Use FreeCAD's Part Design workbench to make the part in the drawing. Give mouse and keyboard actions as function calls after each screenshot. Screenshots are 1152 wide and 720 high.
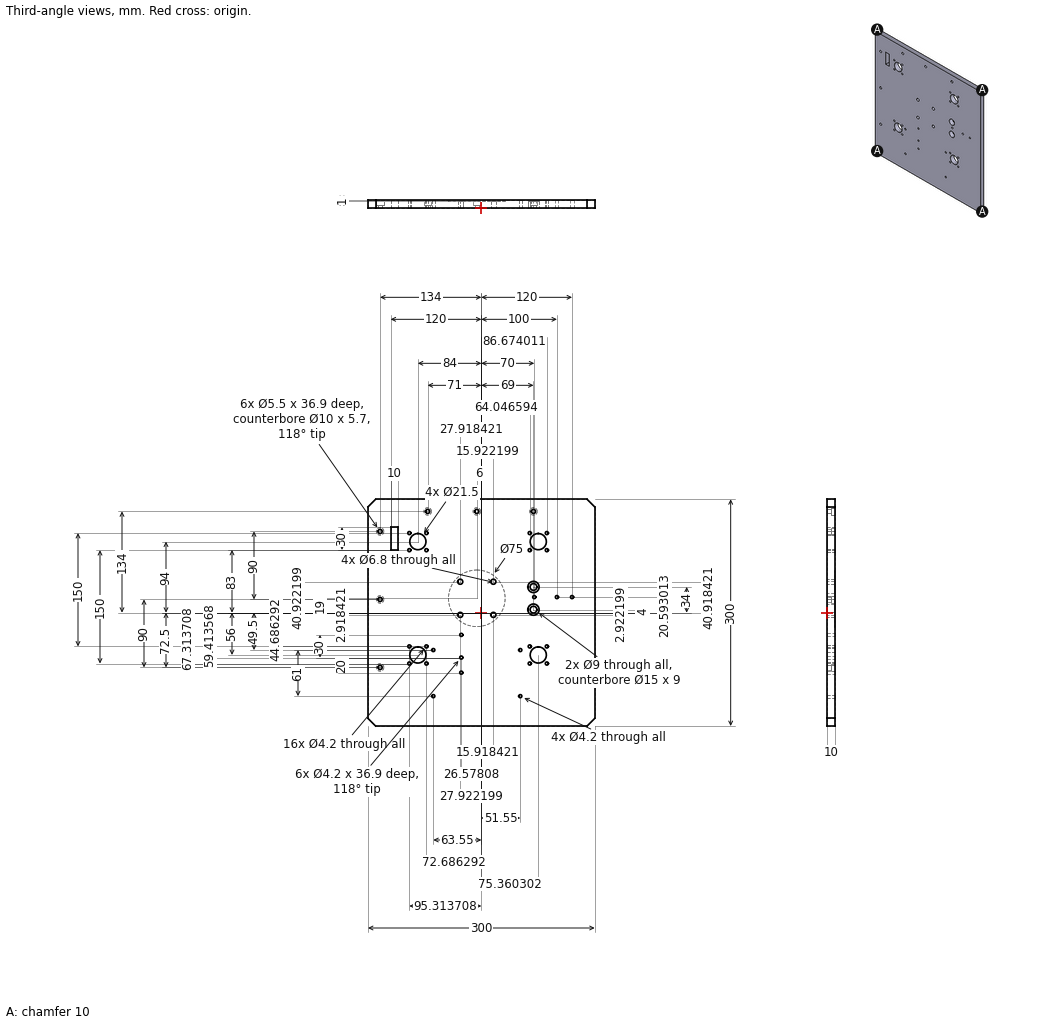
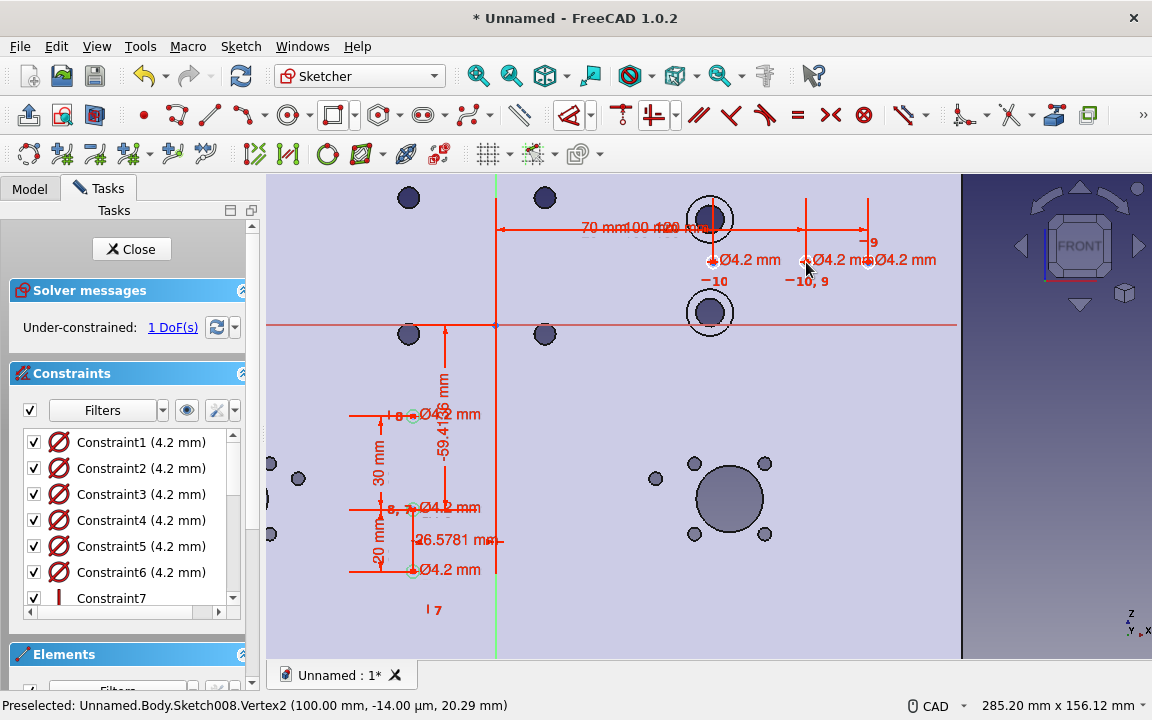
click(590, 116)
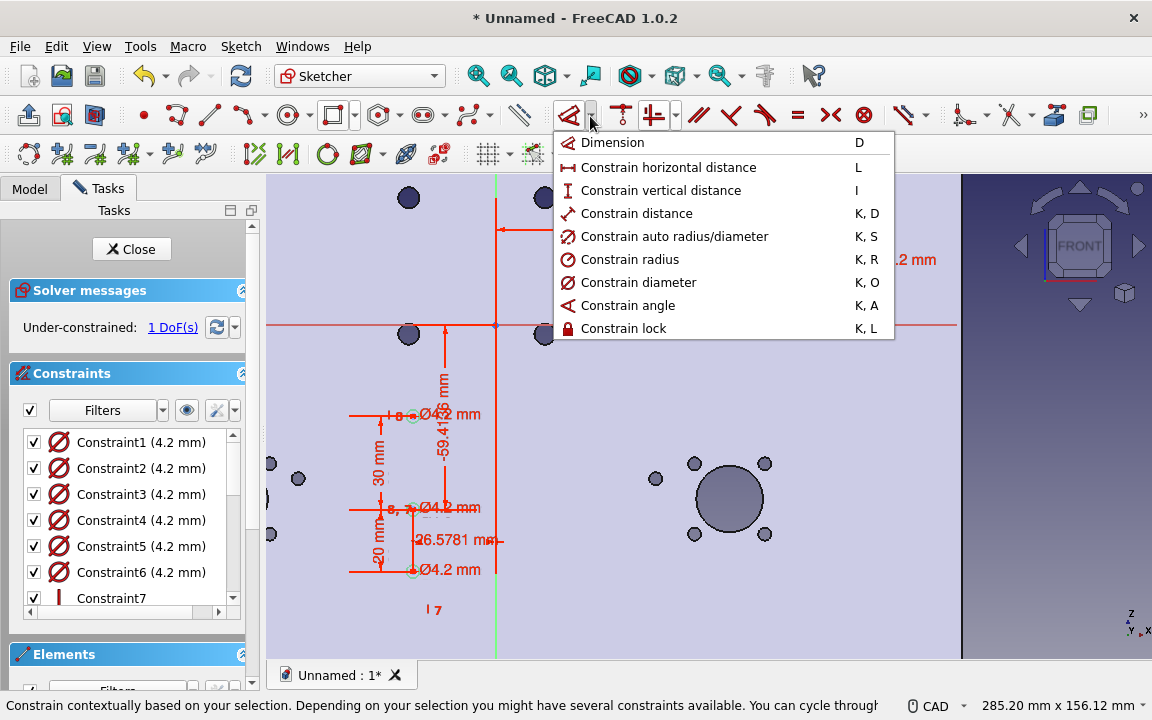
click(724, 190)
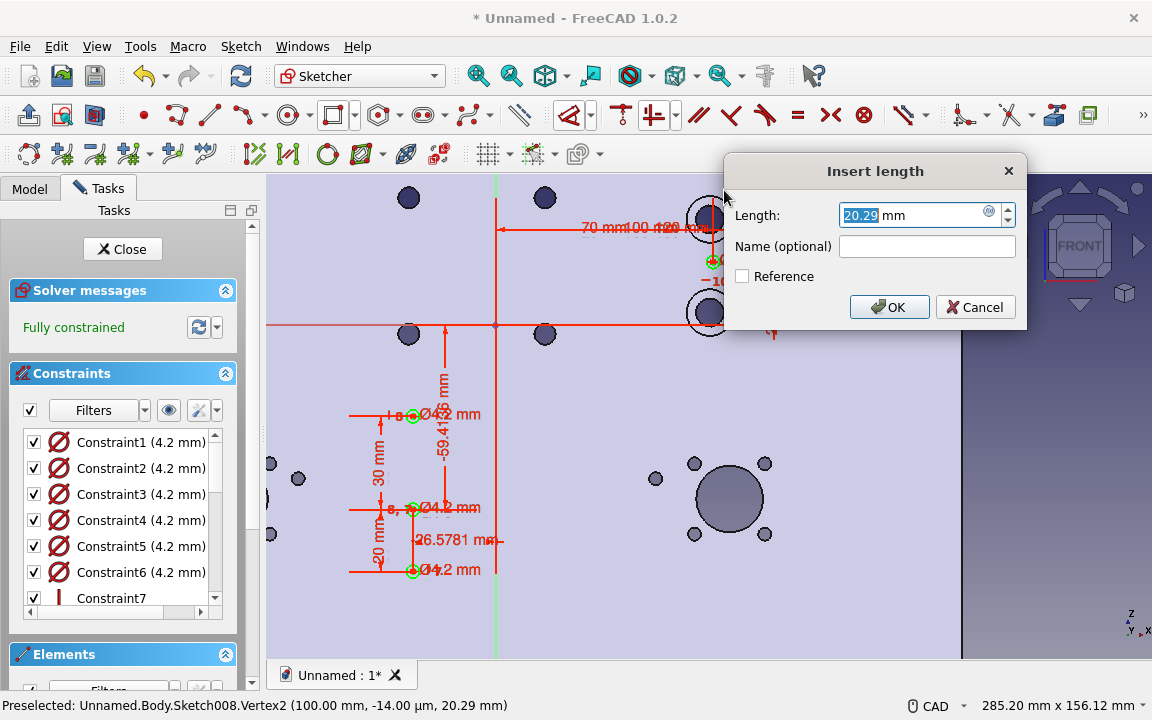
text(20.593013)
key(Return)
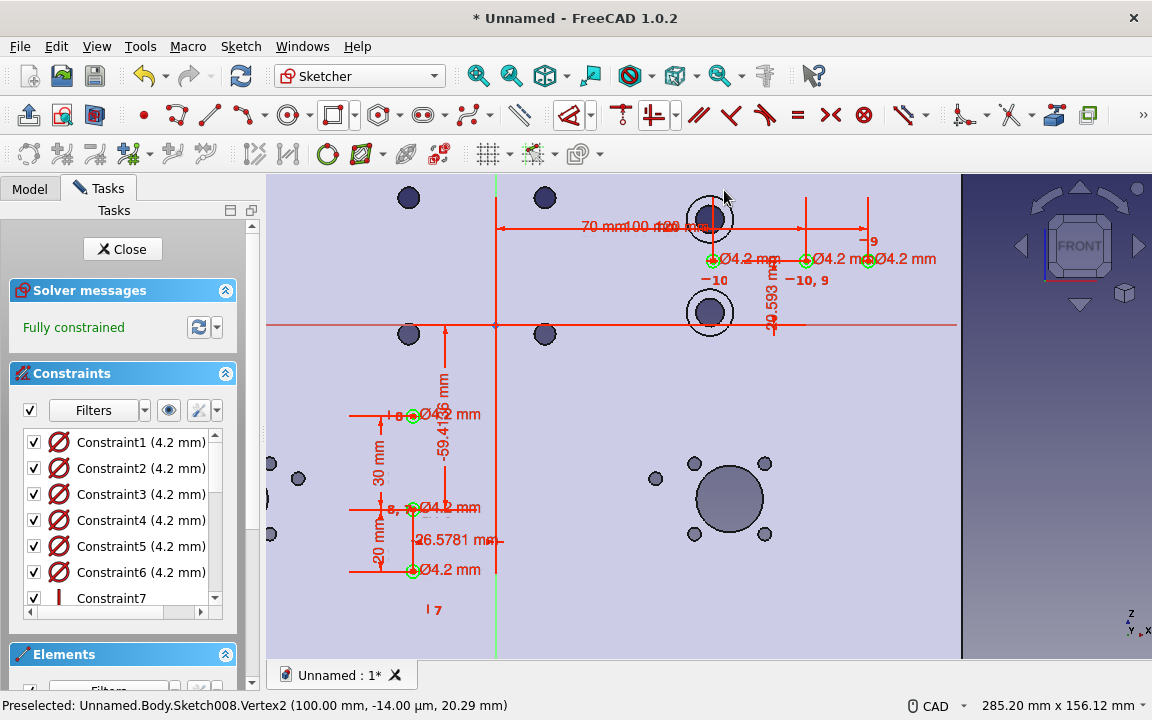
click(123, 249)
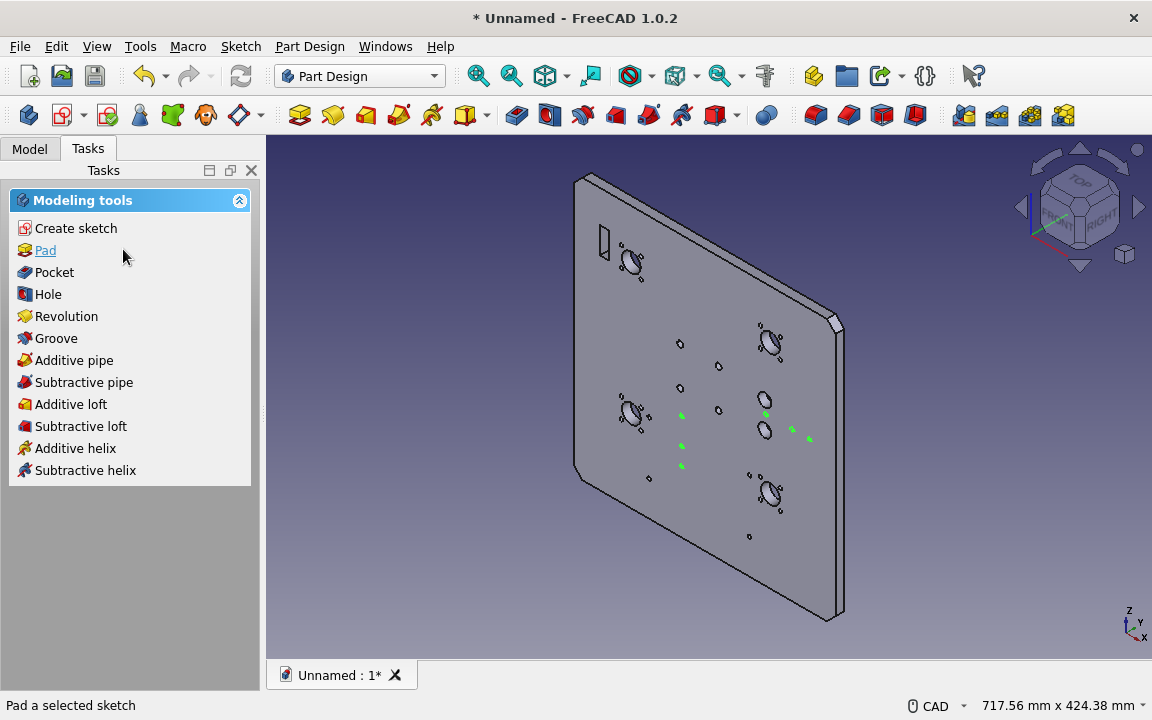
click(550, 116)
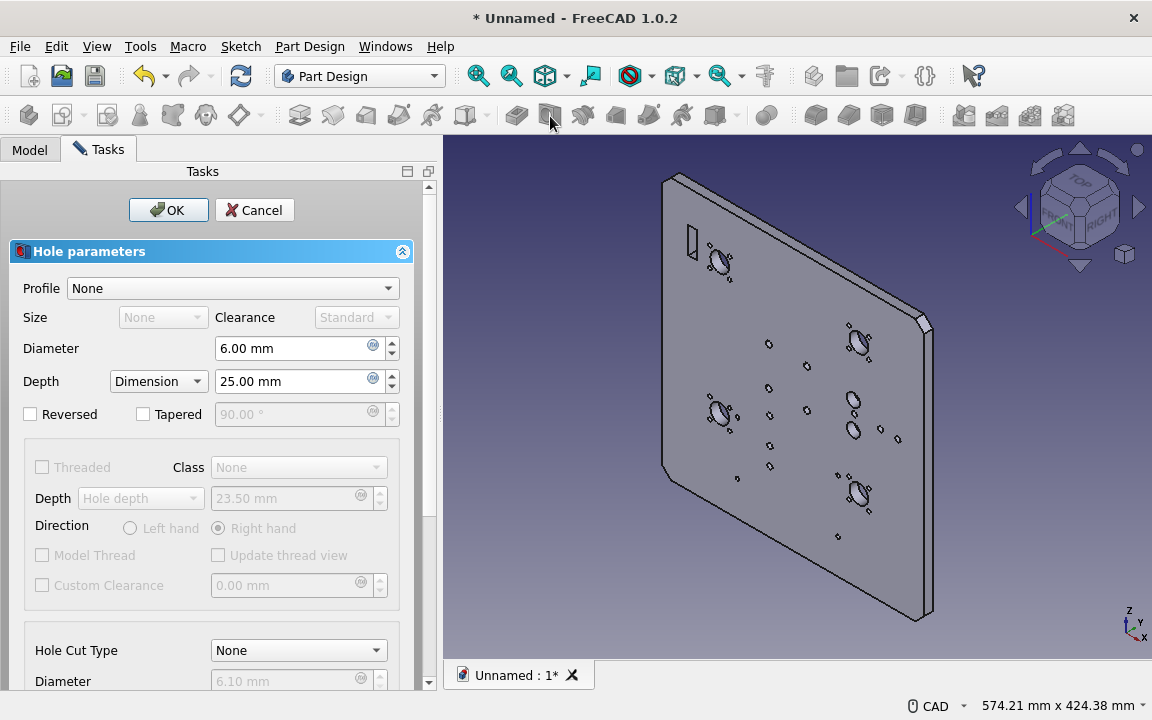
triple_click(300, 348)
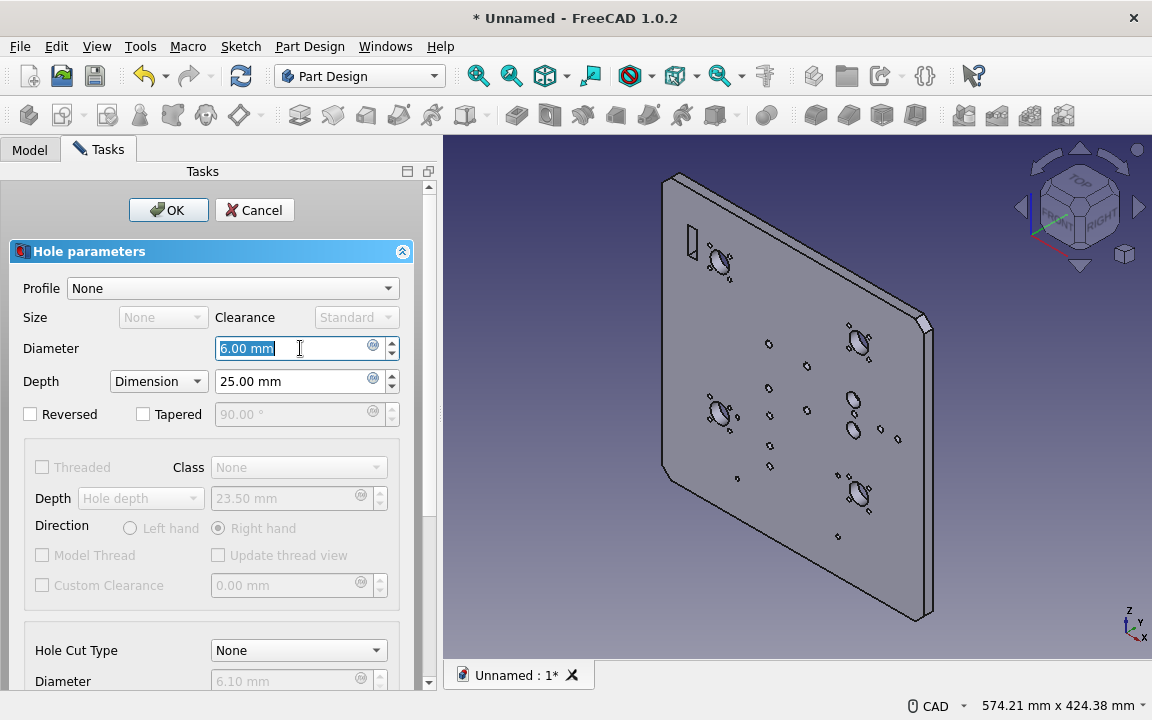
text(4.2)
key(Tab)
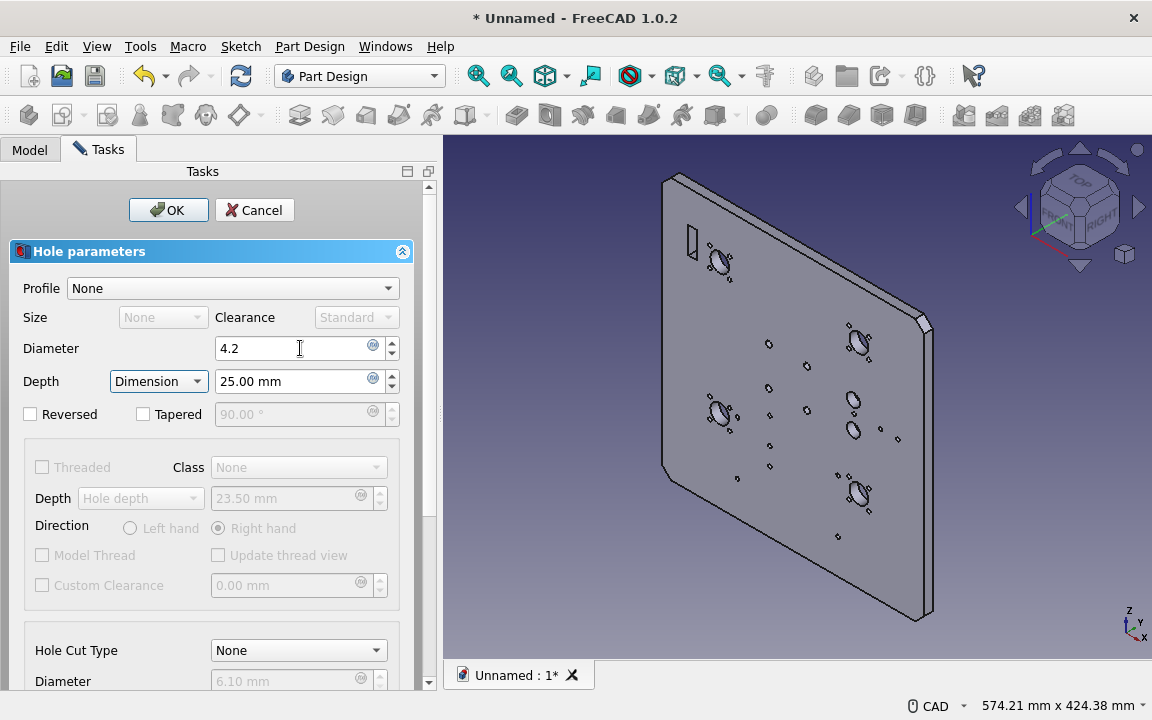
triple_click(300, 382)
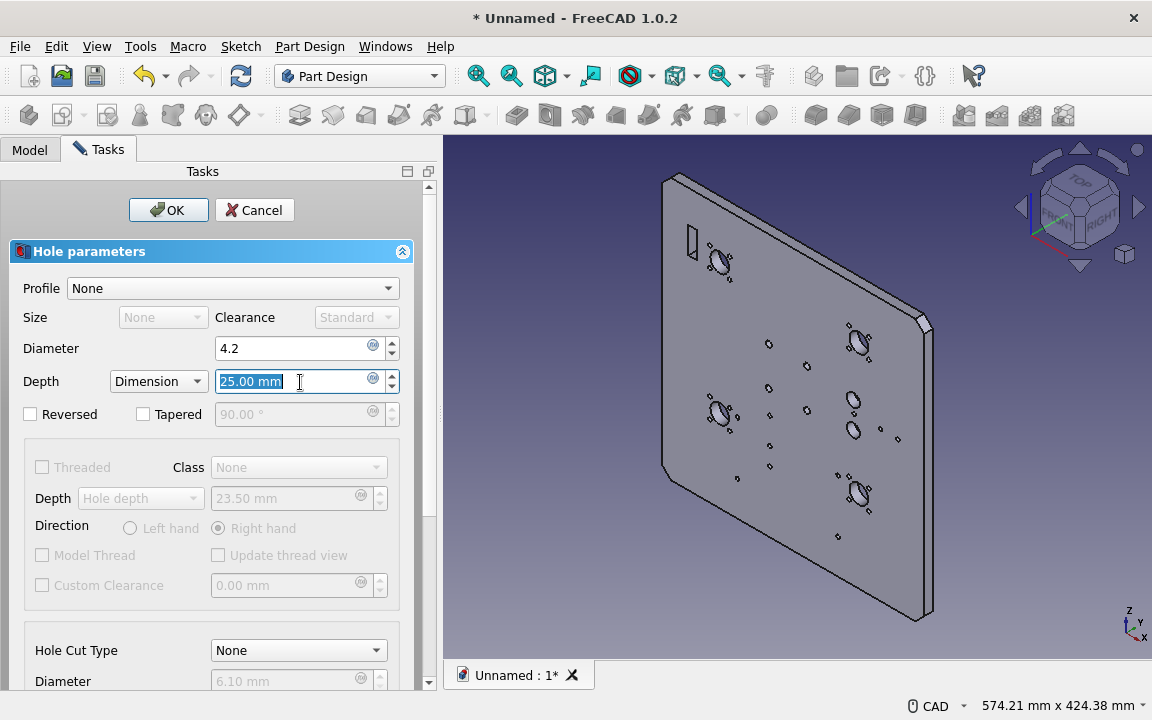
text(36.9)
key(Tab)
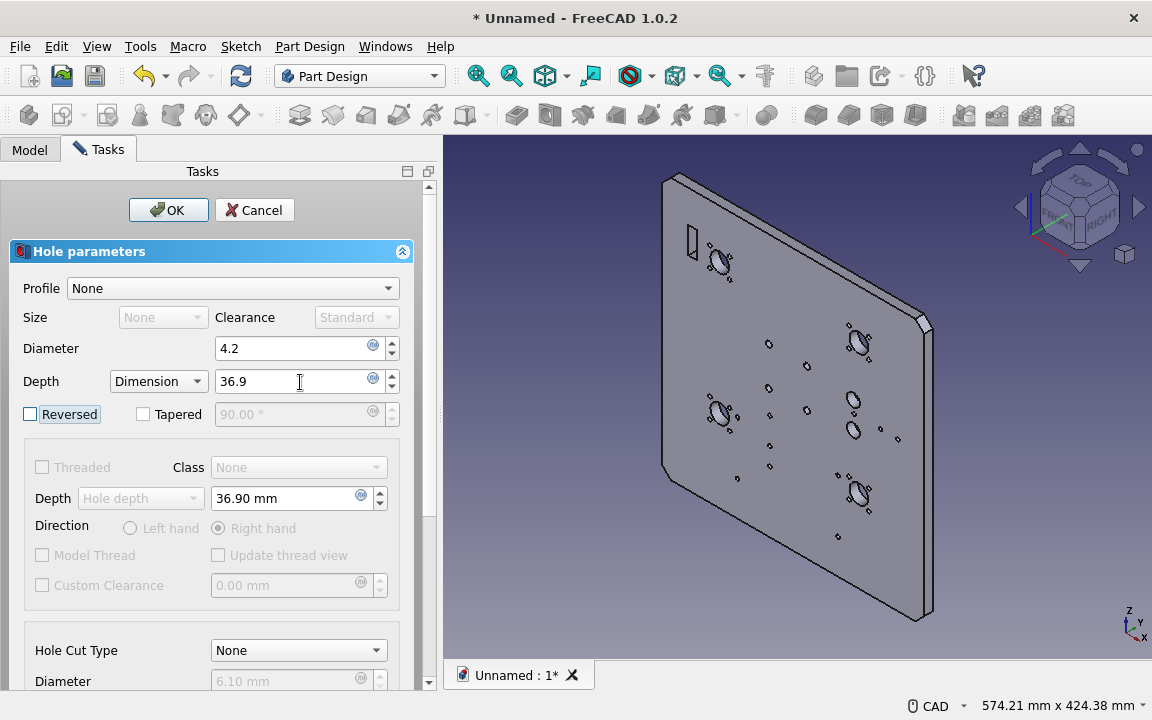
click(169, 210)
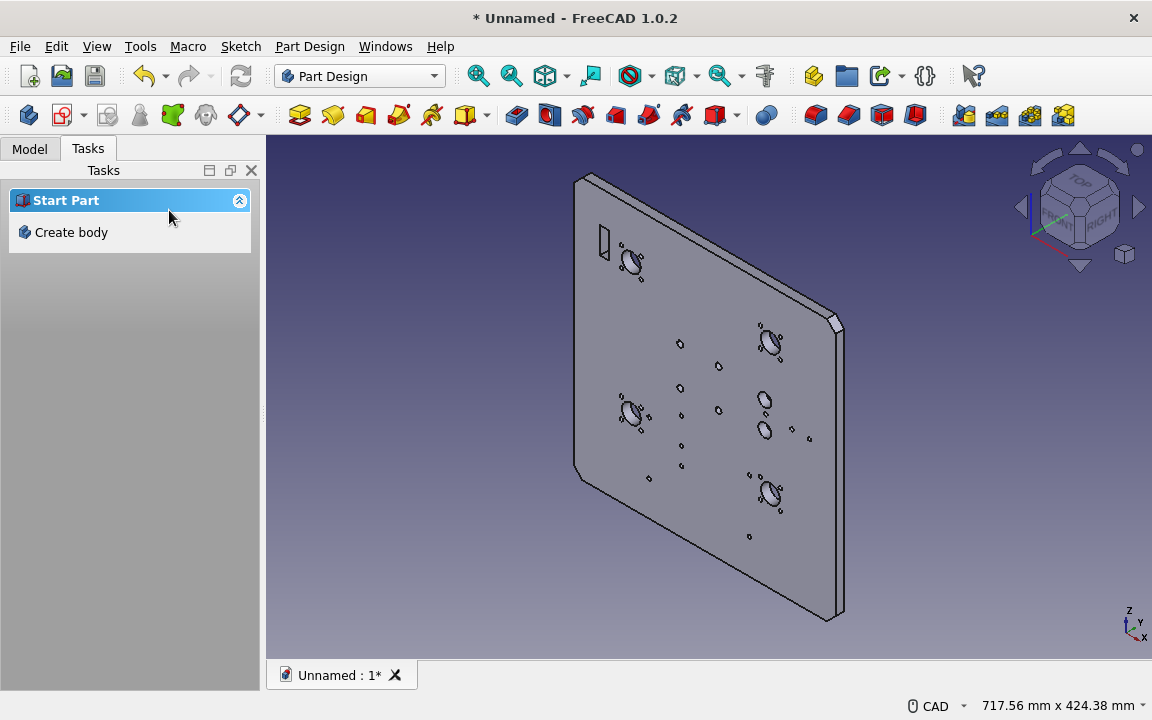
key(4)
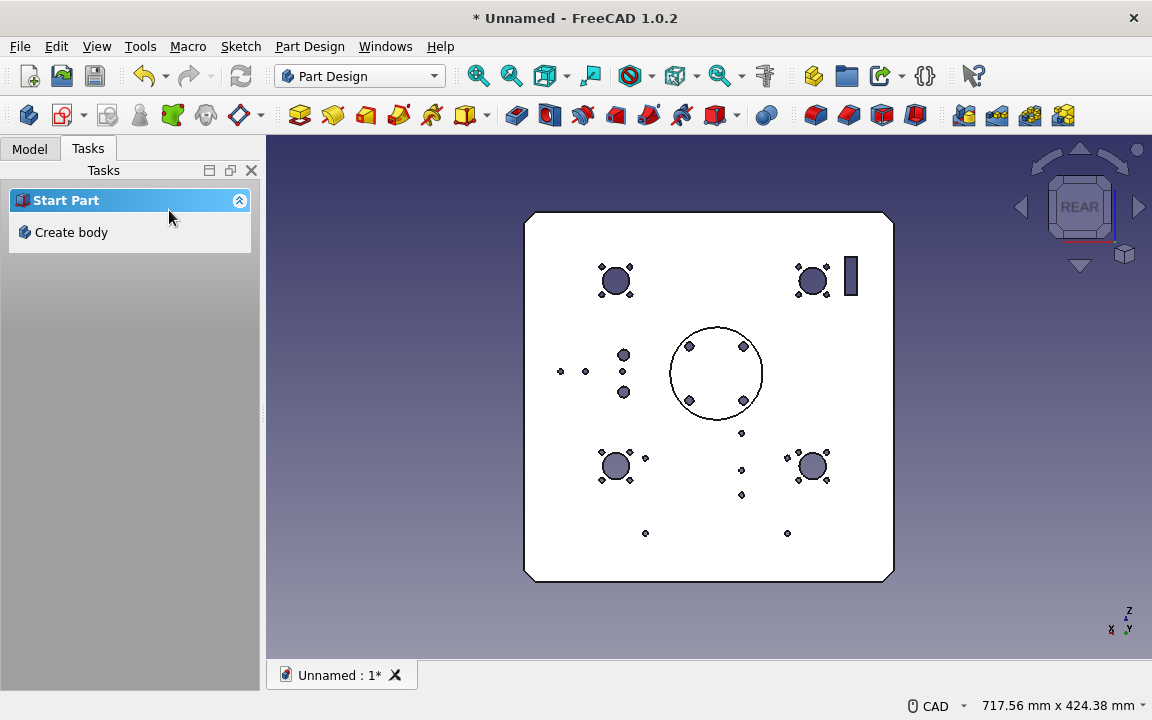
click(815, 396)